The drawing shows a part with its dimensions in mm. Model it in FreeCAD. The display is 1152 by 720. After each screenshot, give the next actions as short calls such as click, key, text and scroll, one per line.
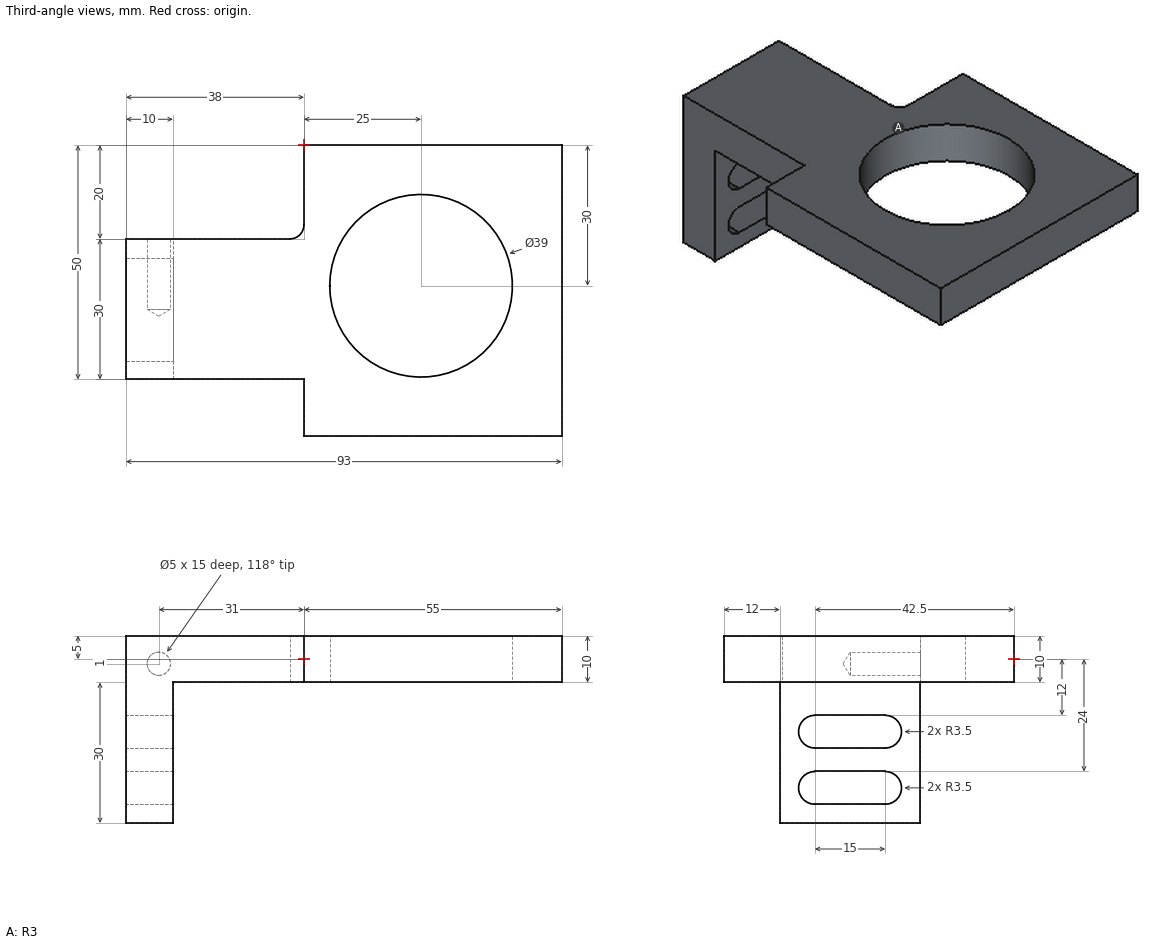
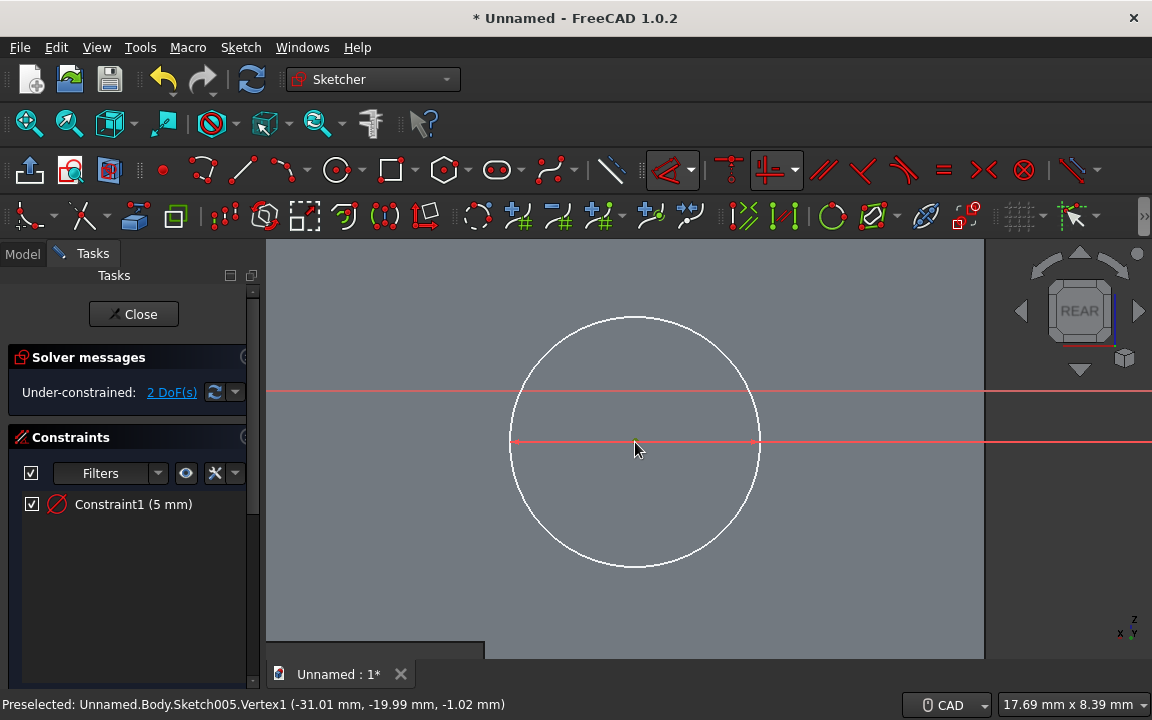
click(694, 170)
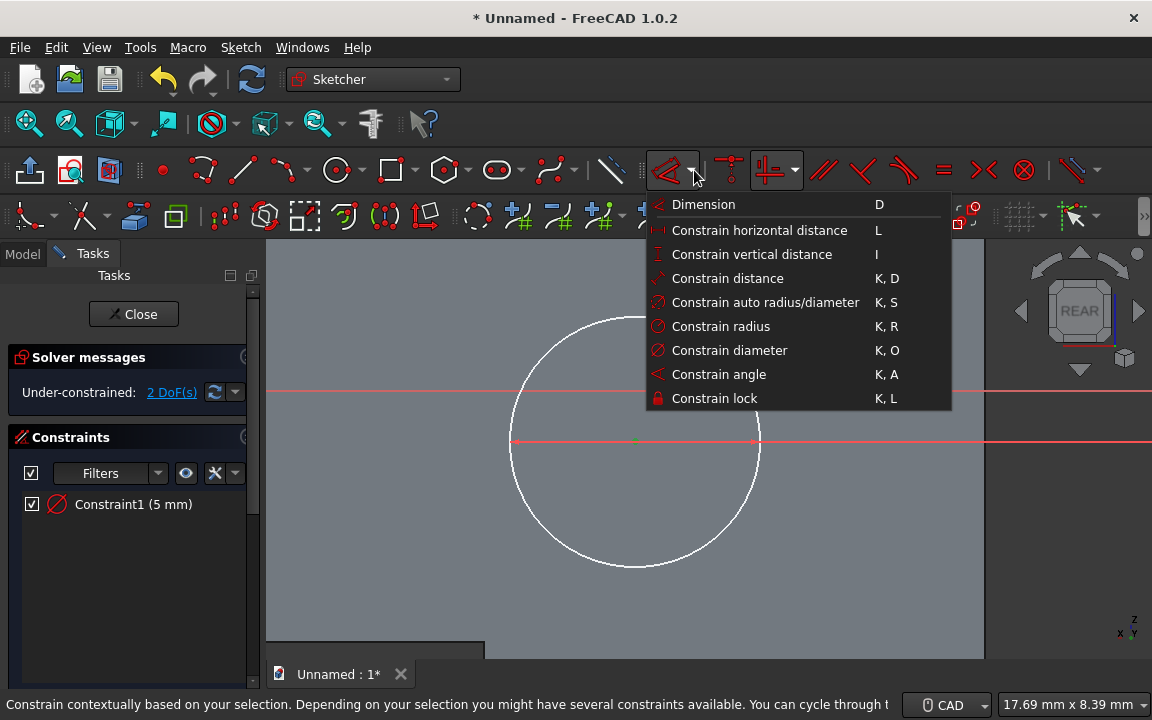
click(799, 254)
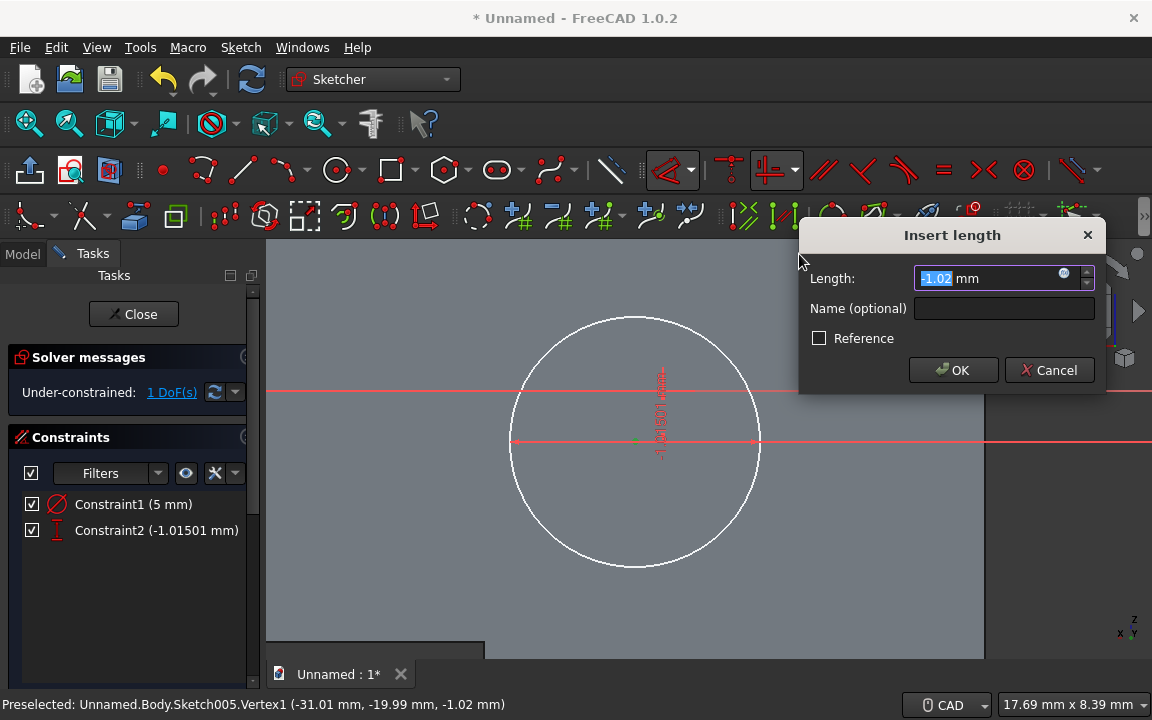
text(-1)
key(Return)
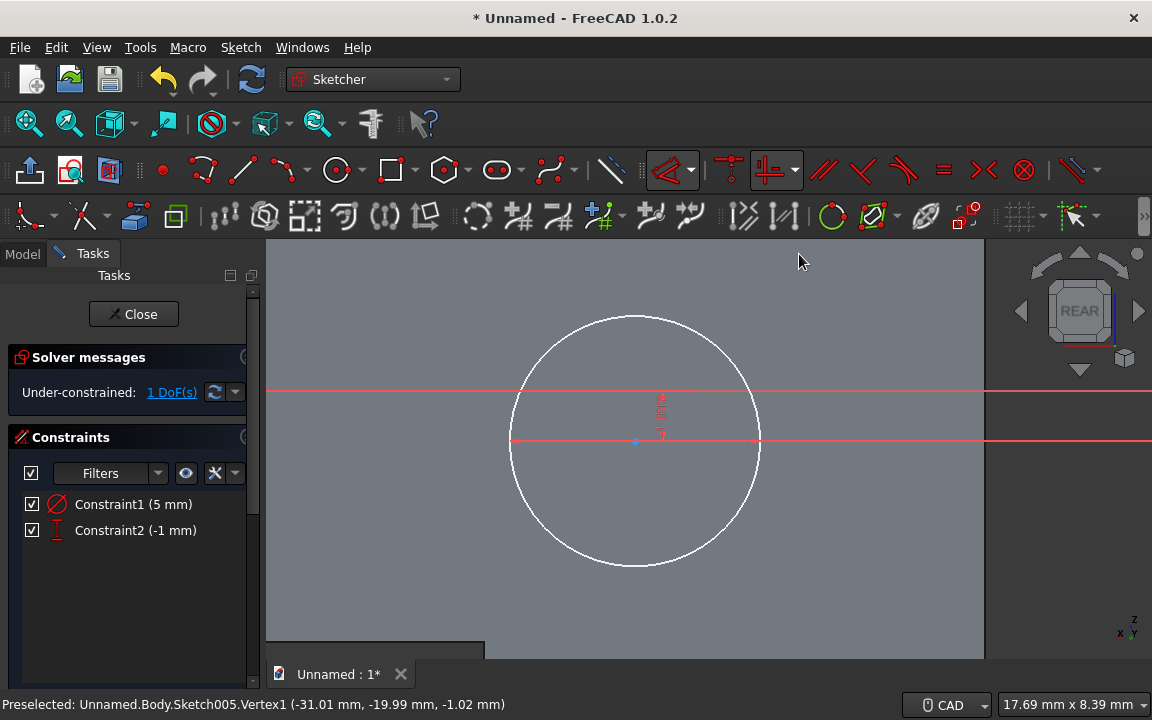
click(635, 441)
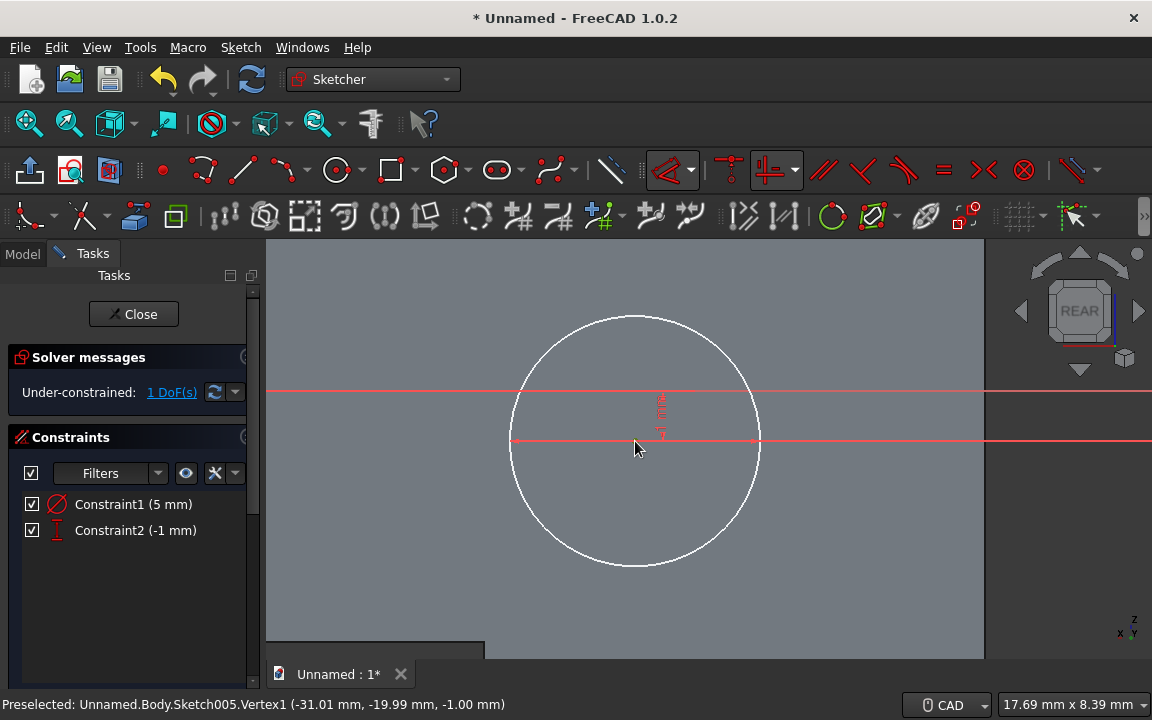
key(l)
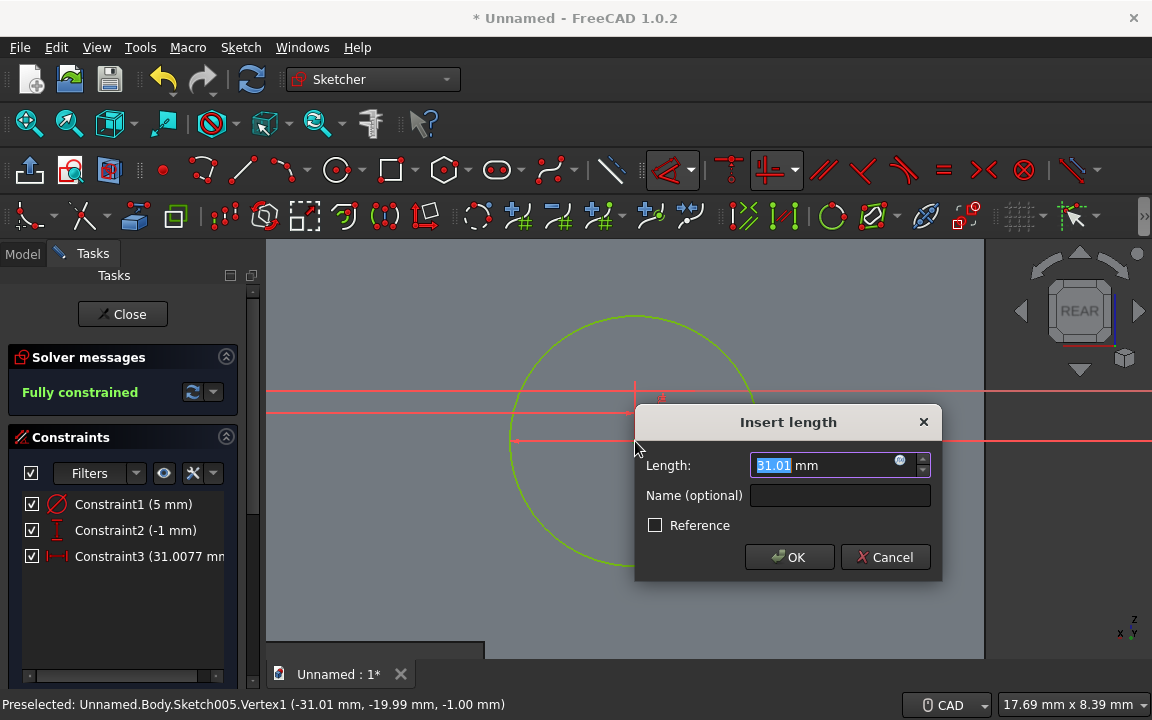
text(31)
key(Return)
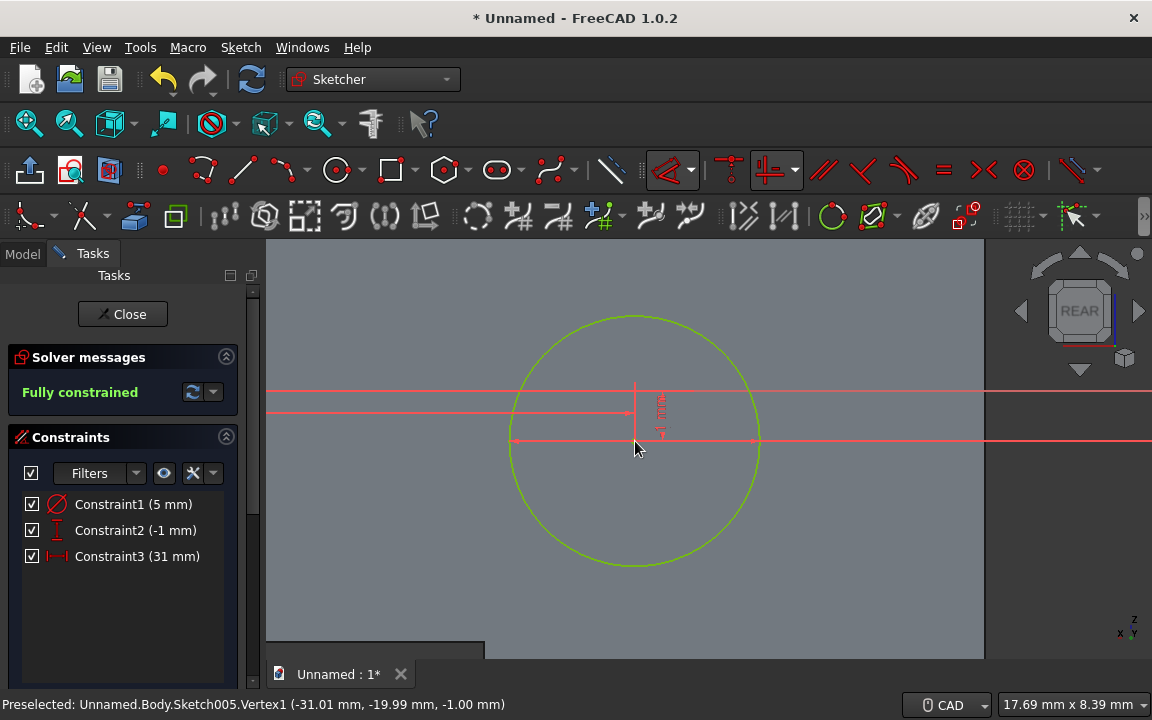
click(123, 314)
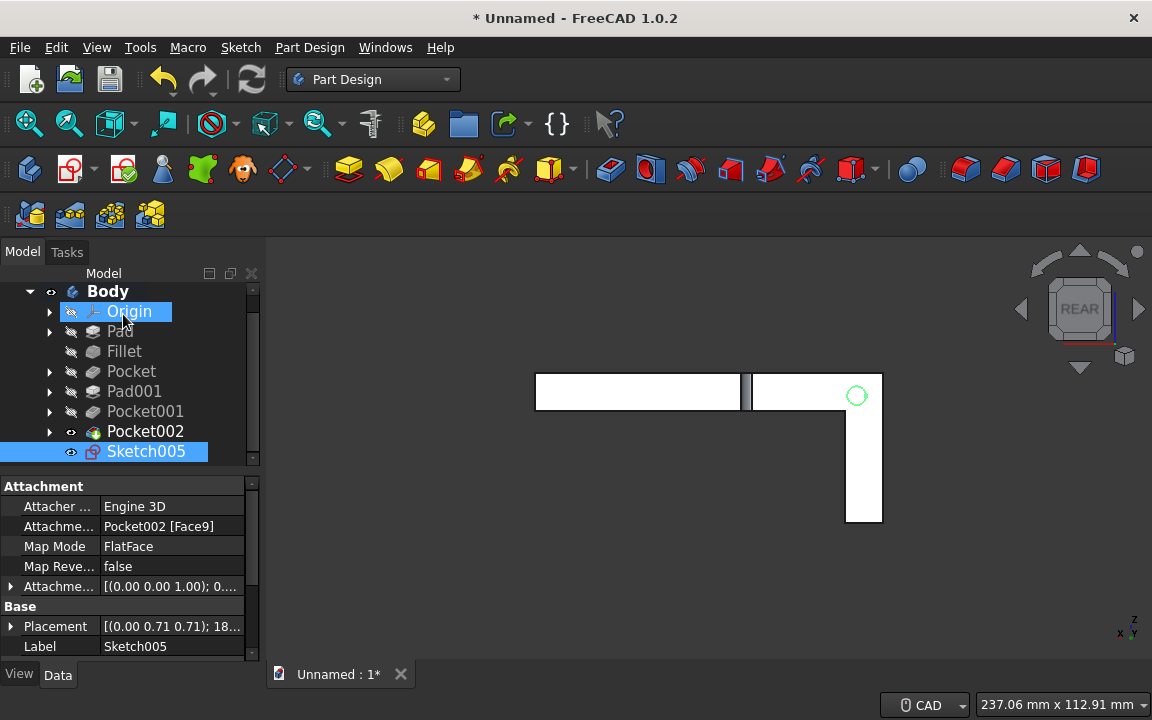
click(652, 170)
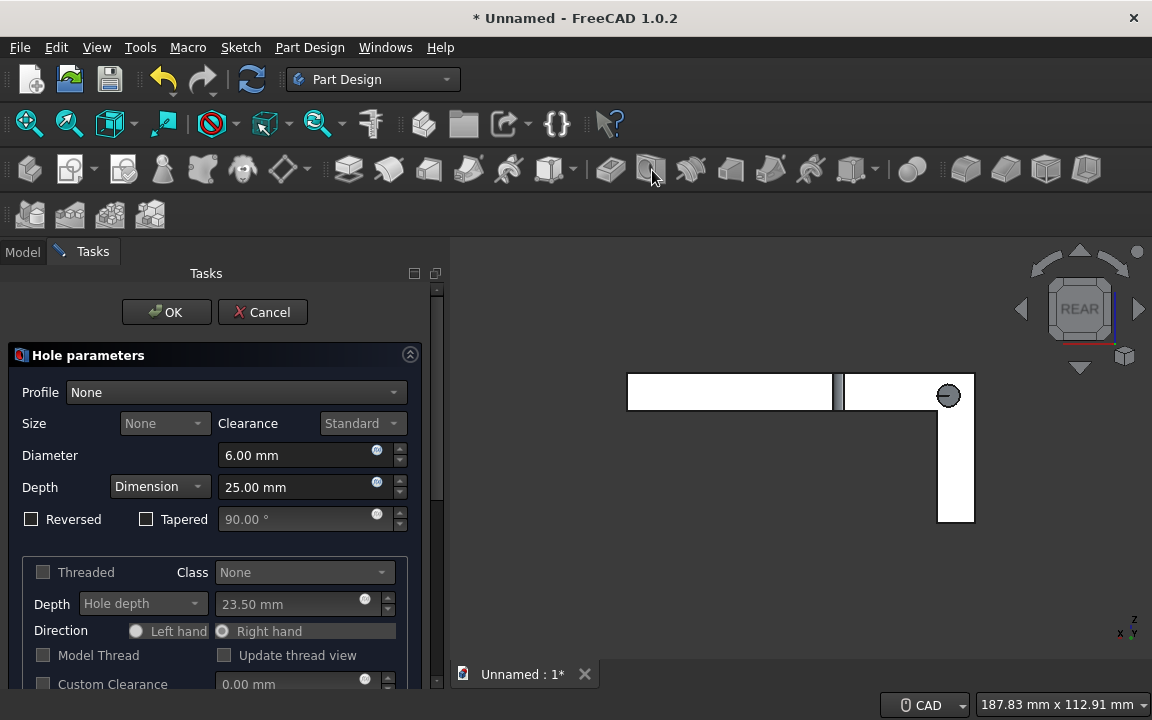
triple_click(305, 455)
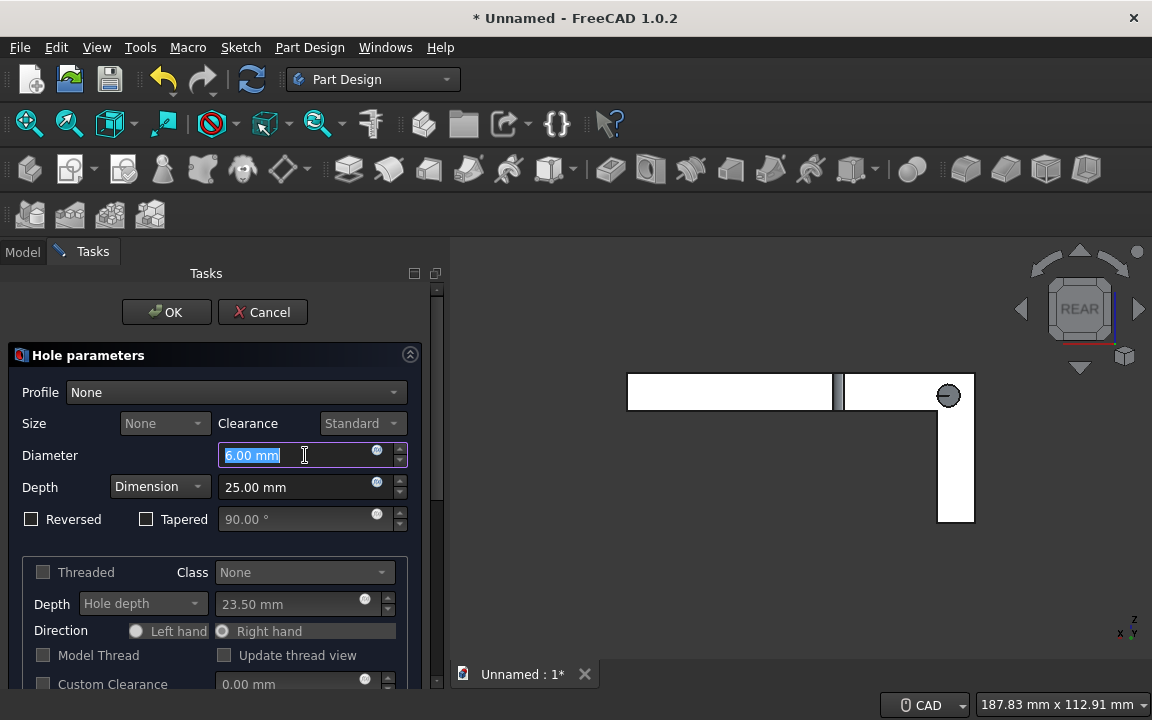
text(5)
key(Tab)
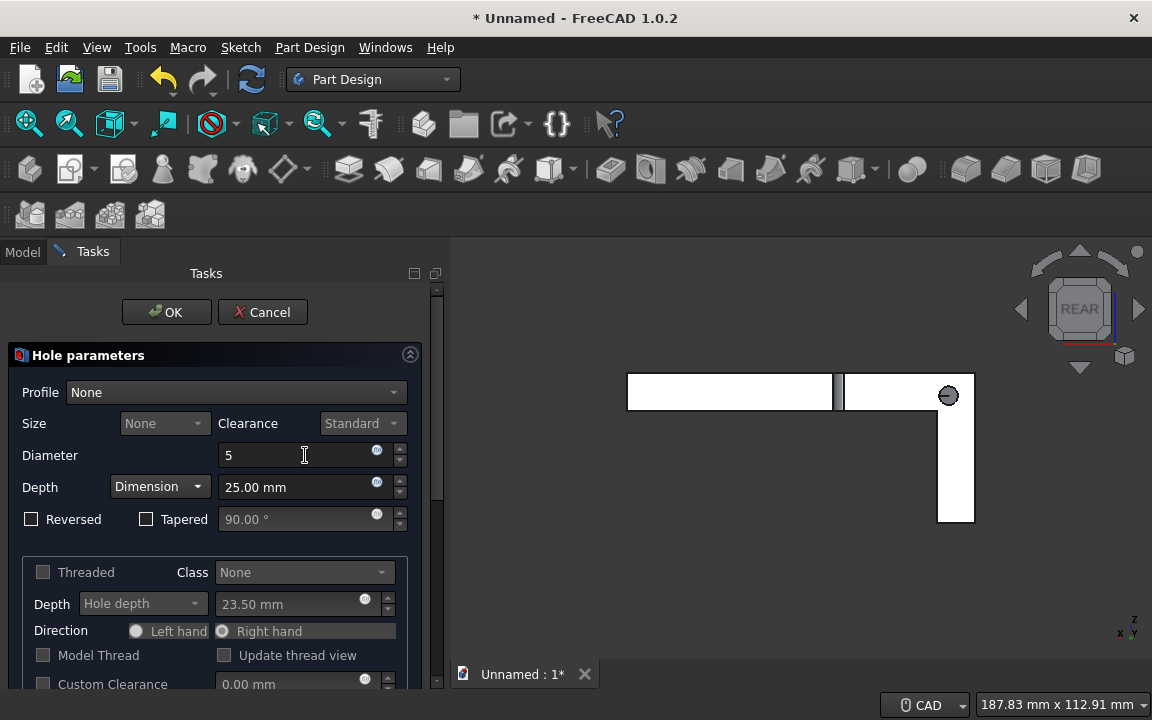
triple_click(305, 487)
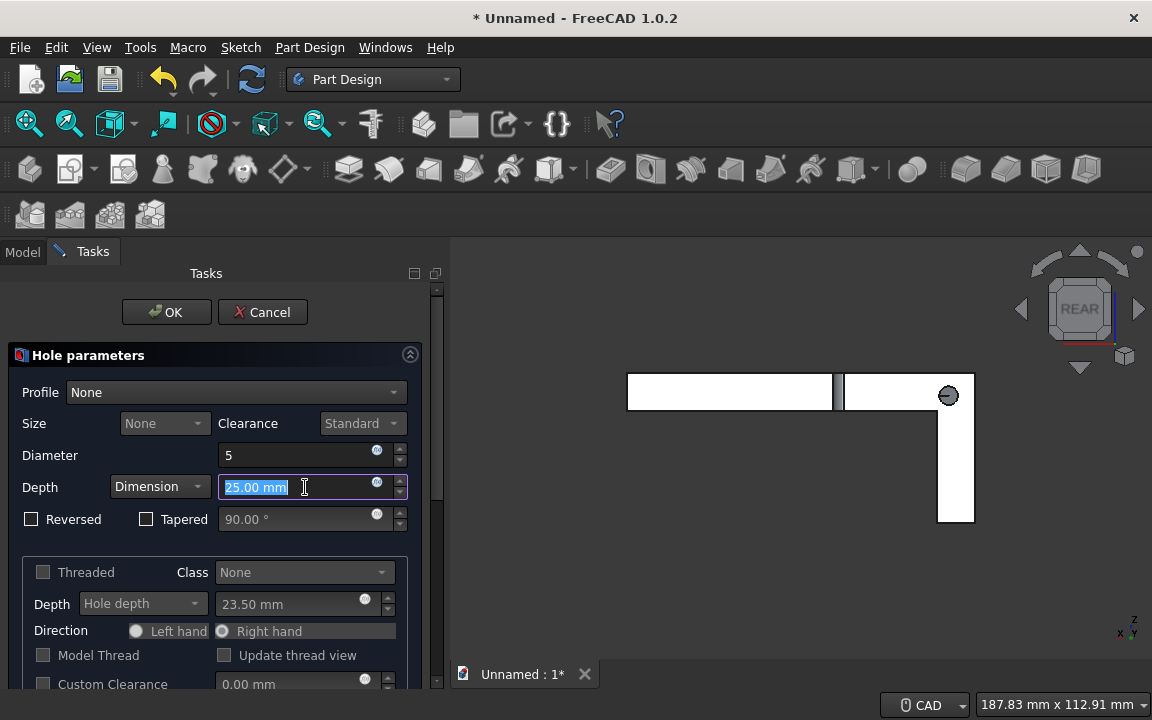
text(15)
key(Tab)